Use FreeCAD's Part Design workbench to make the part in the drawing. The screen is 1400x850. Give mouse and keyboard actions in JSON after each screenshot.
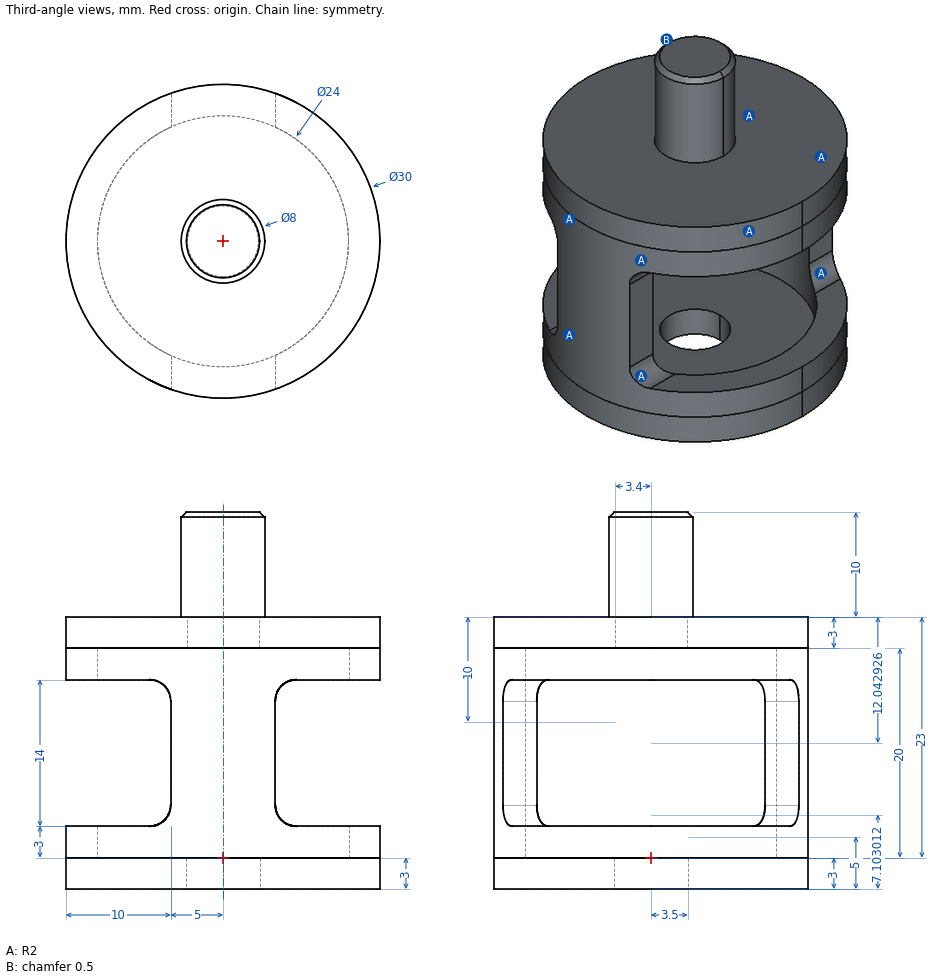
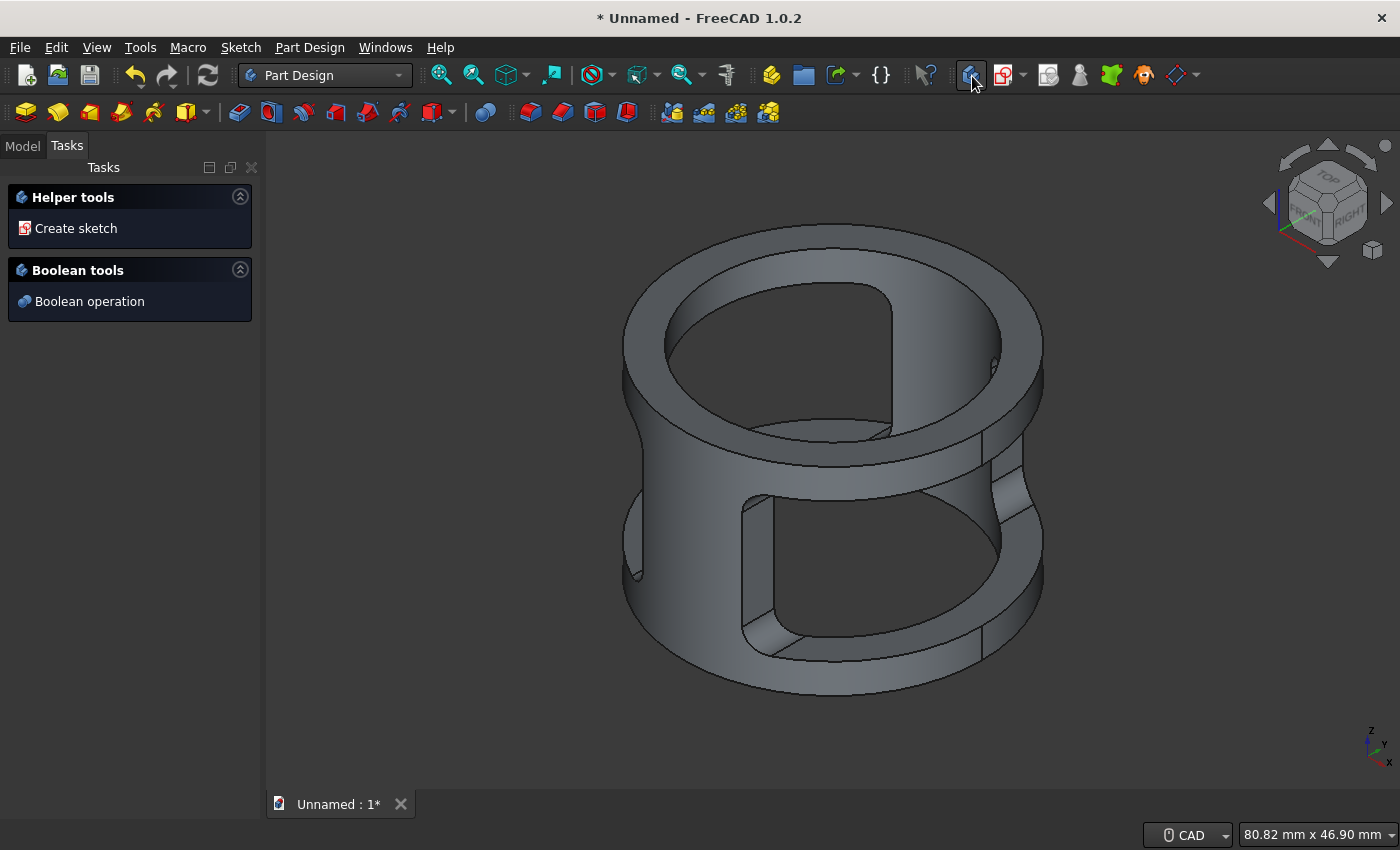
{"action": "left_click", "coordinate": [23, 145]}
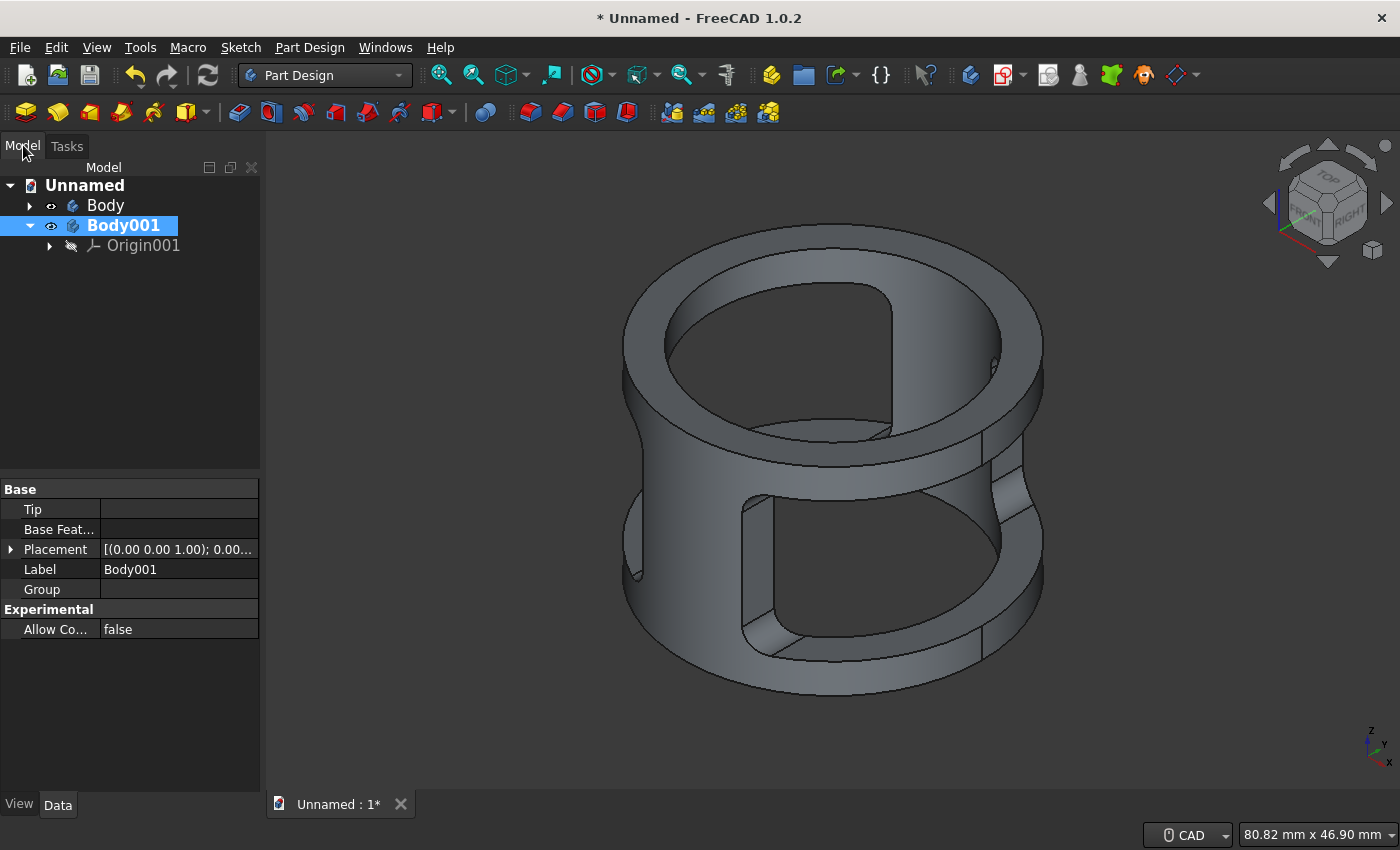
{"action": "left_click", "coordinate": [50, 246]}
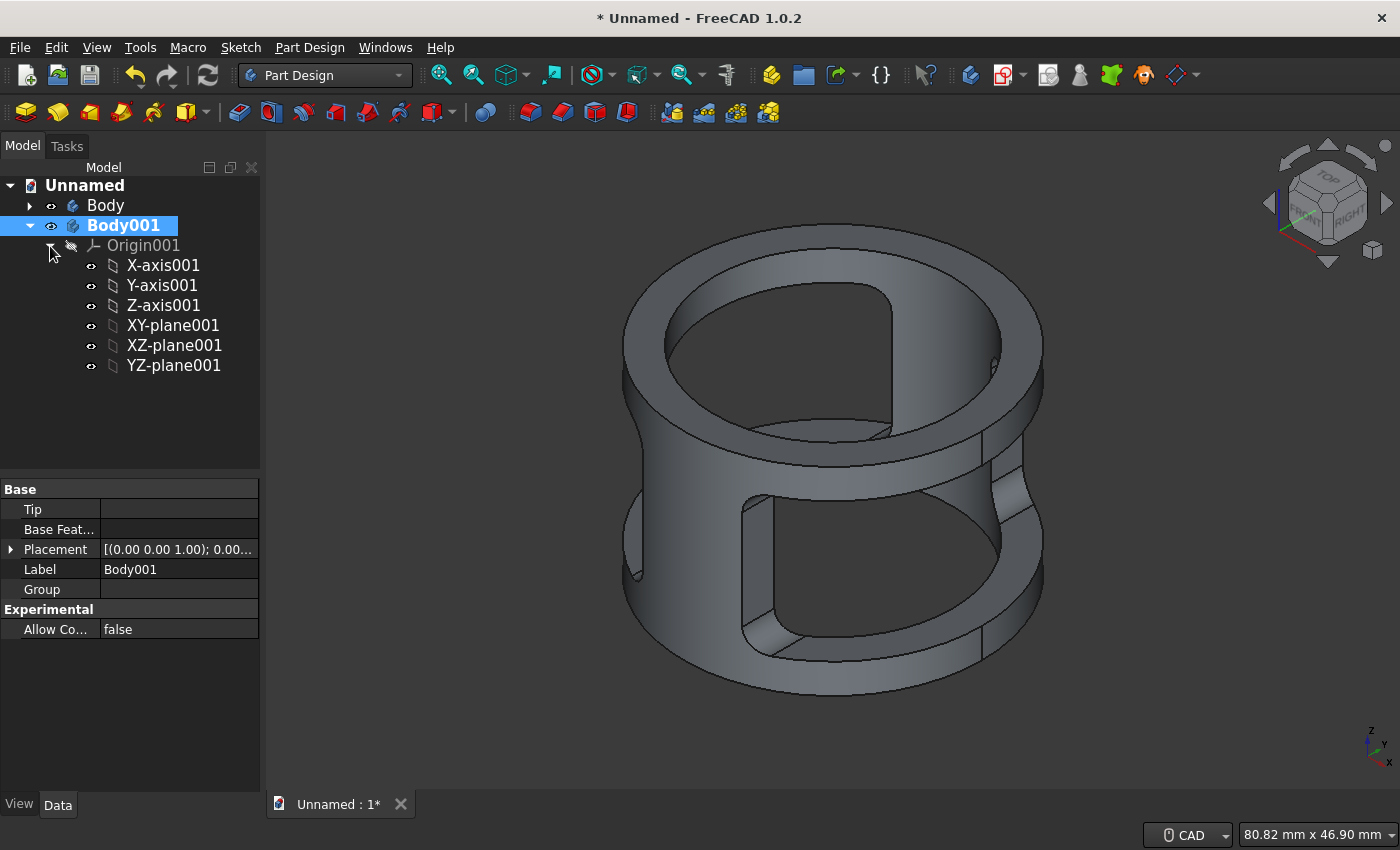
{"action": "left_click", "coordinate": [136, 326]}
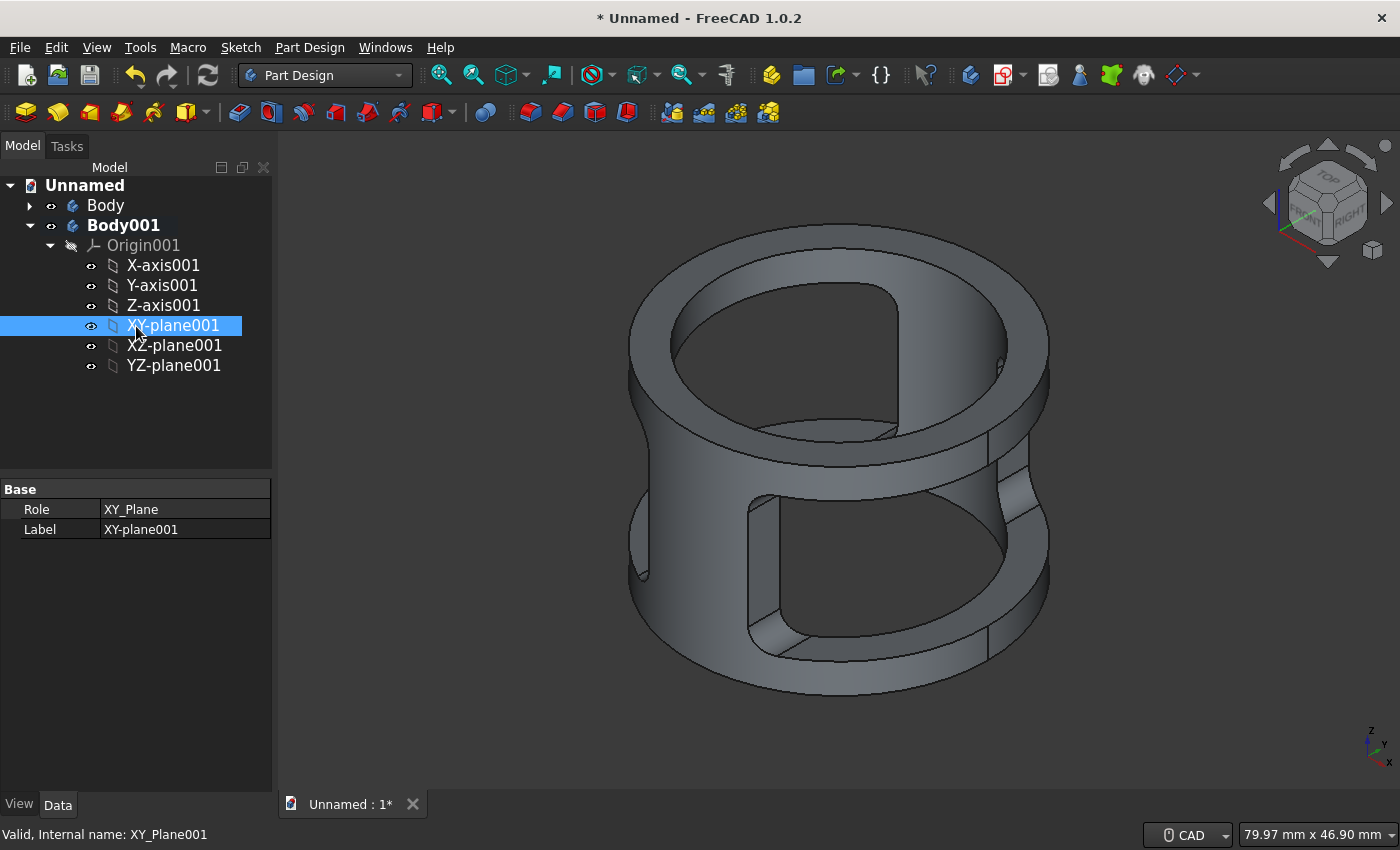
{"action": "left_click", "coordinate": [1176, 76]}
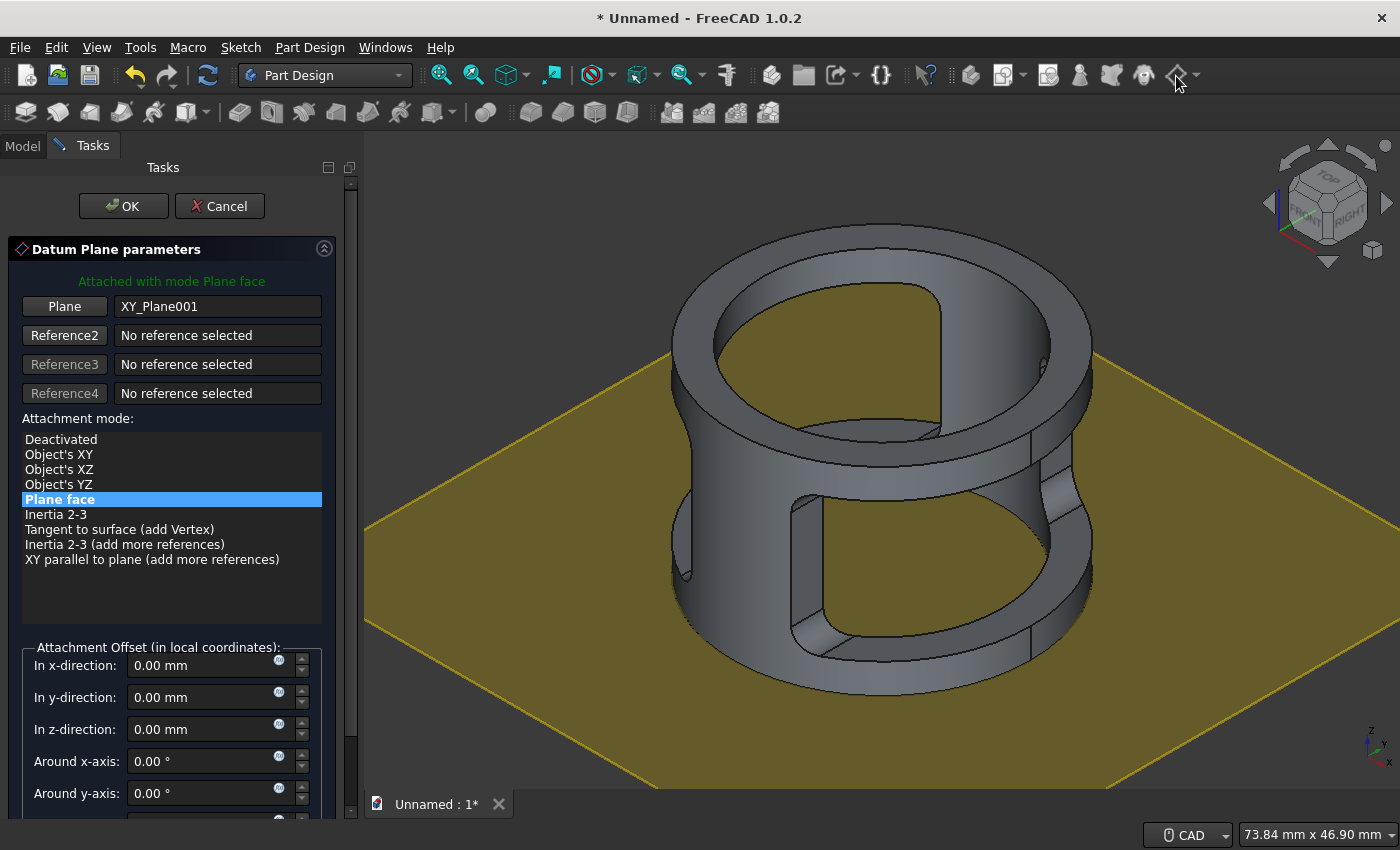
{"action": "triple_click", "coordinate": [210, 729]}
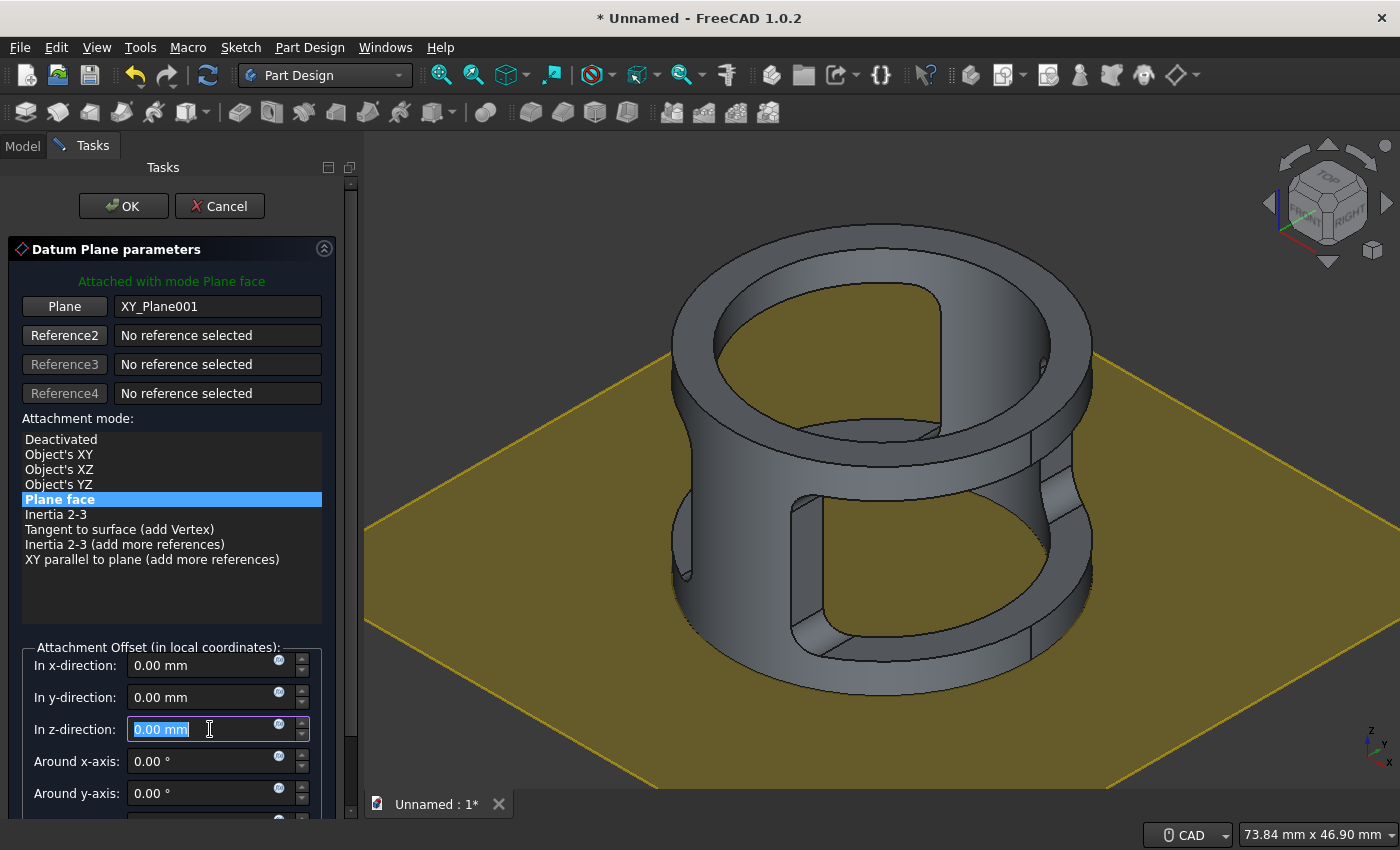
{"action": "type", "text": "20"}
{"action": "key", "text": "Tab"}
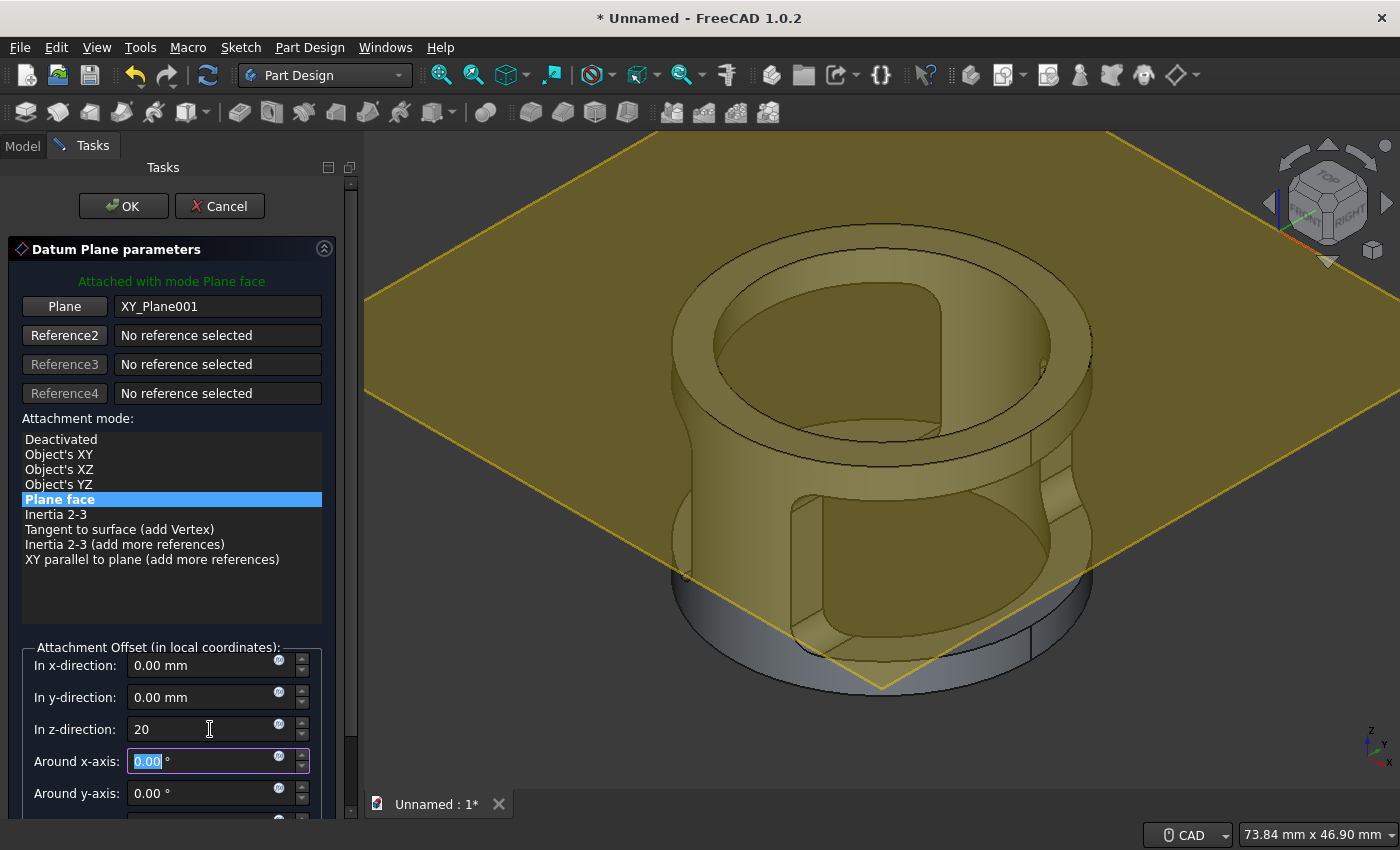
{"action": "left_click", "coordinate": [124, 206]}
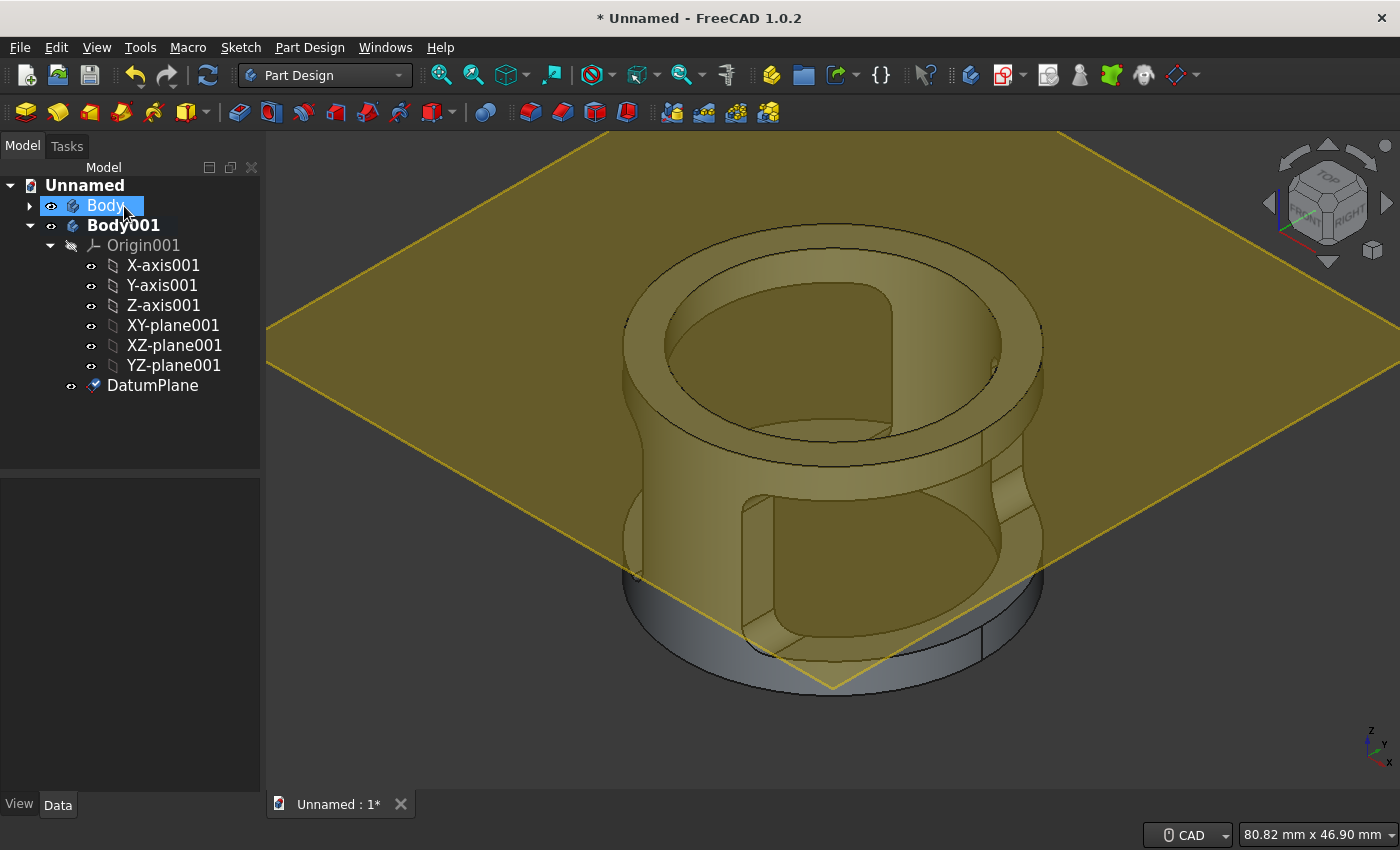
{"action": "left_click", "coordinate": [116, 386]}